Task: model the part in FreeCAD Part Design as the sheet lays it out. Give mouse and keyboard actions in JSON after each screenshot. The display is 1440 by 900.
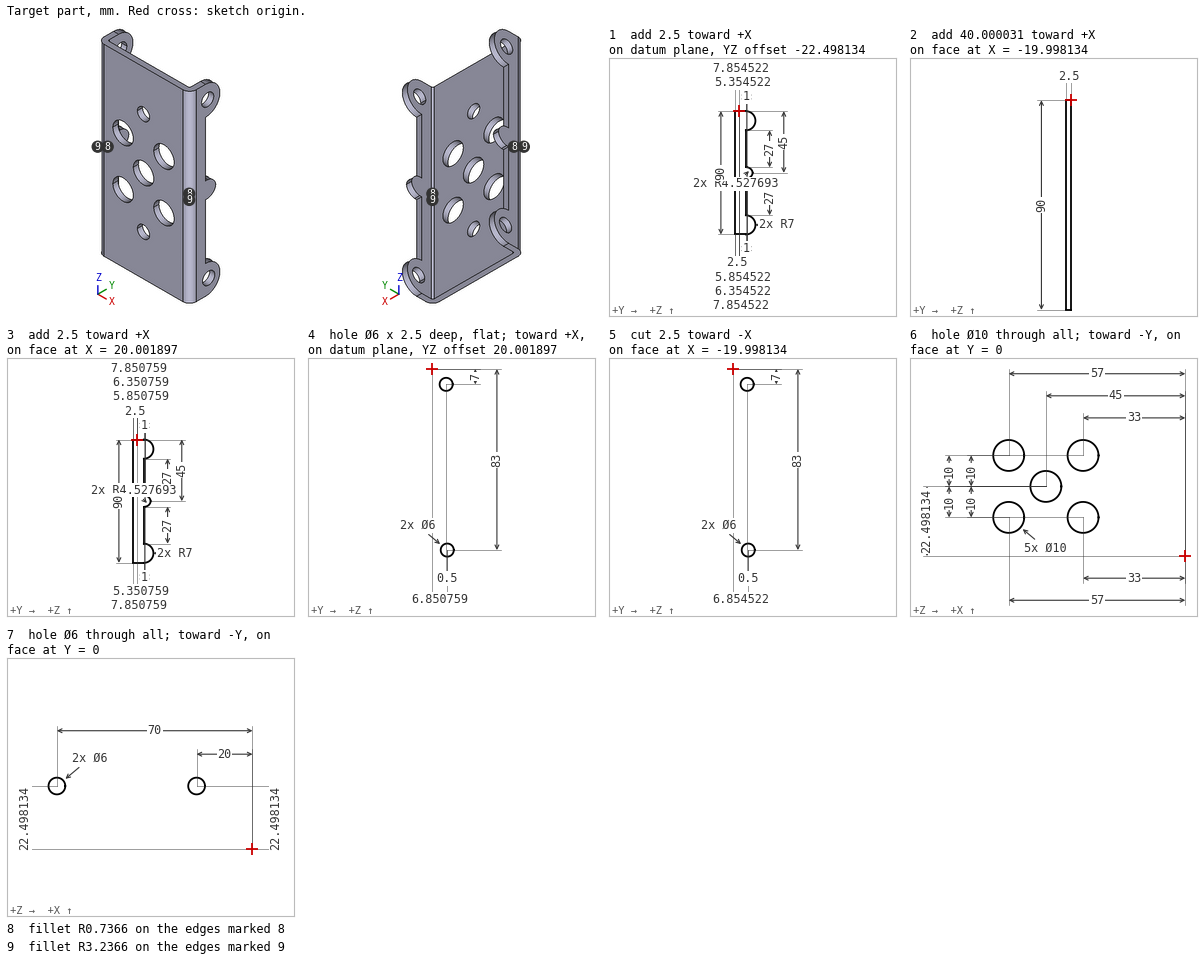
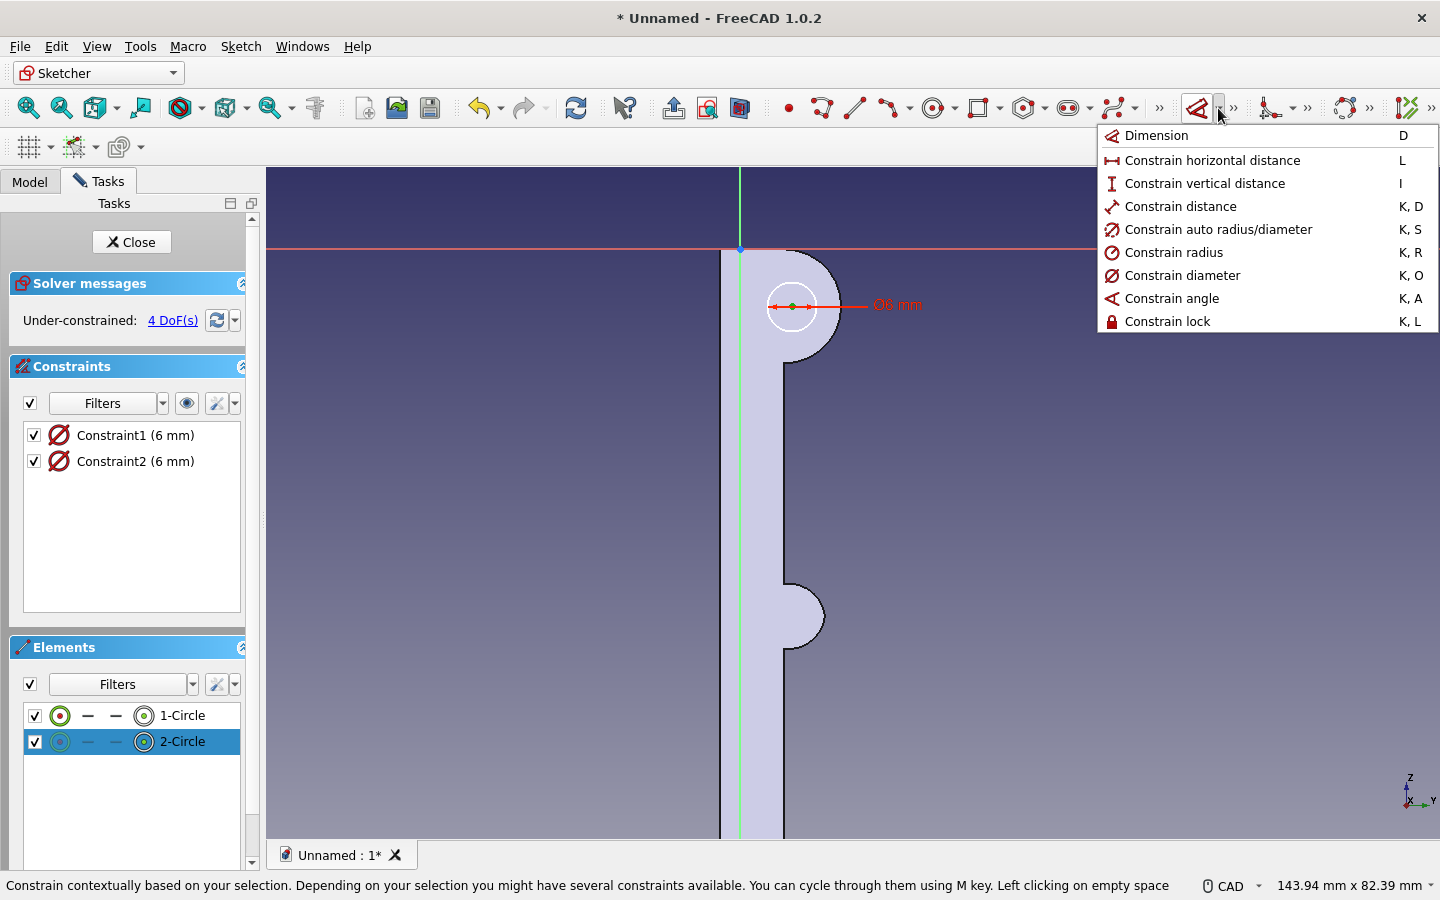
{"action": "left_click", "coordinate": [1268, 184]}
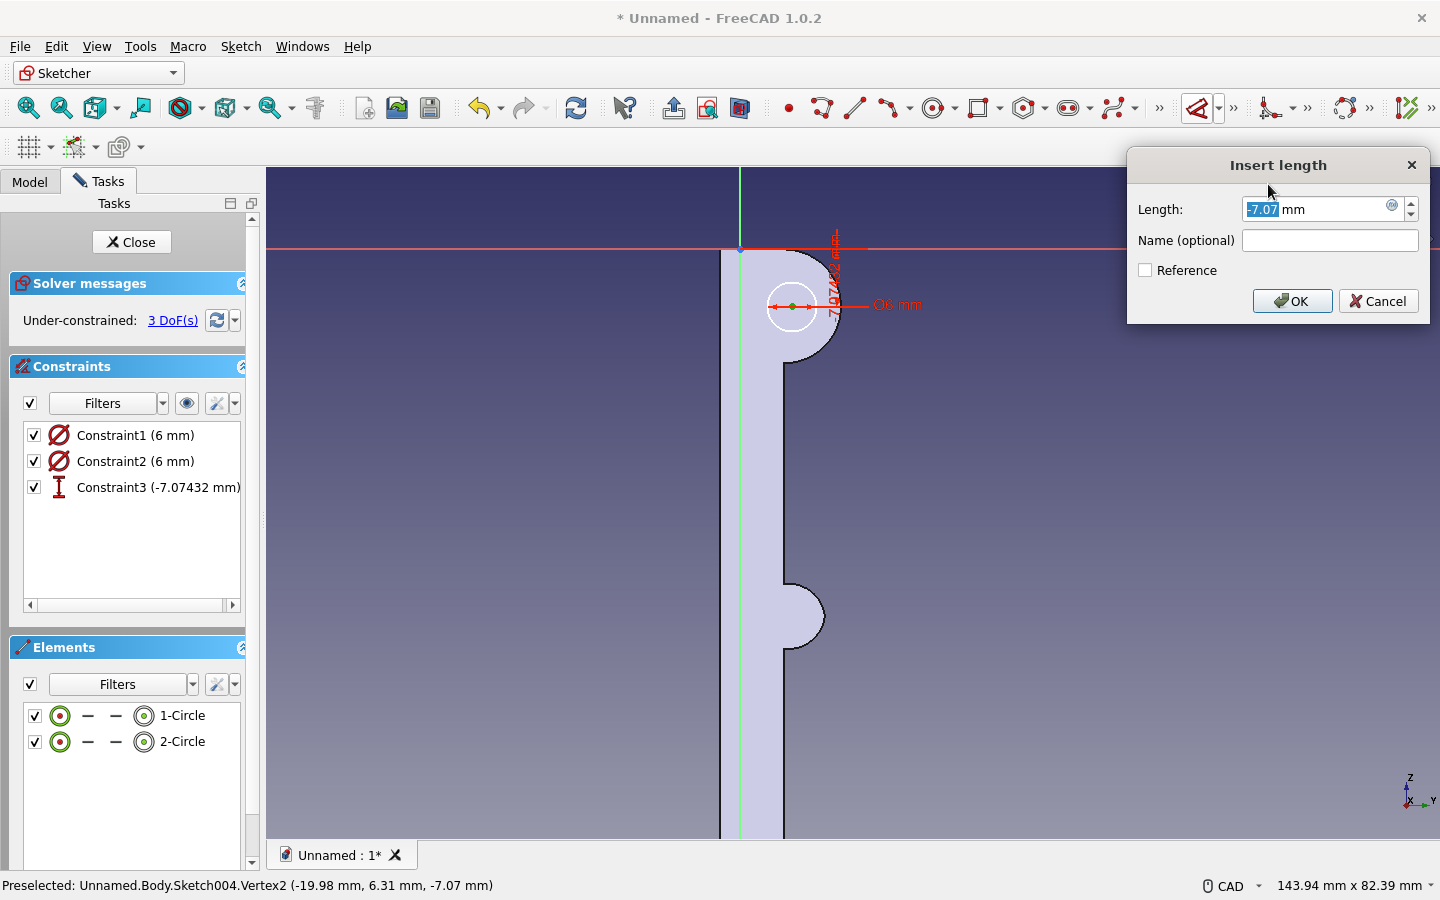
{"action": "type", "text": "-7"}
{"action": "key", "text": "Return"}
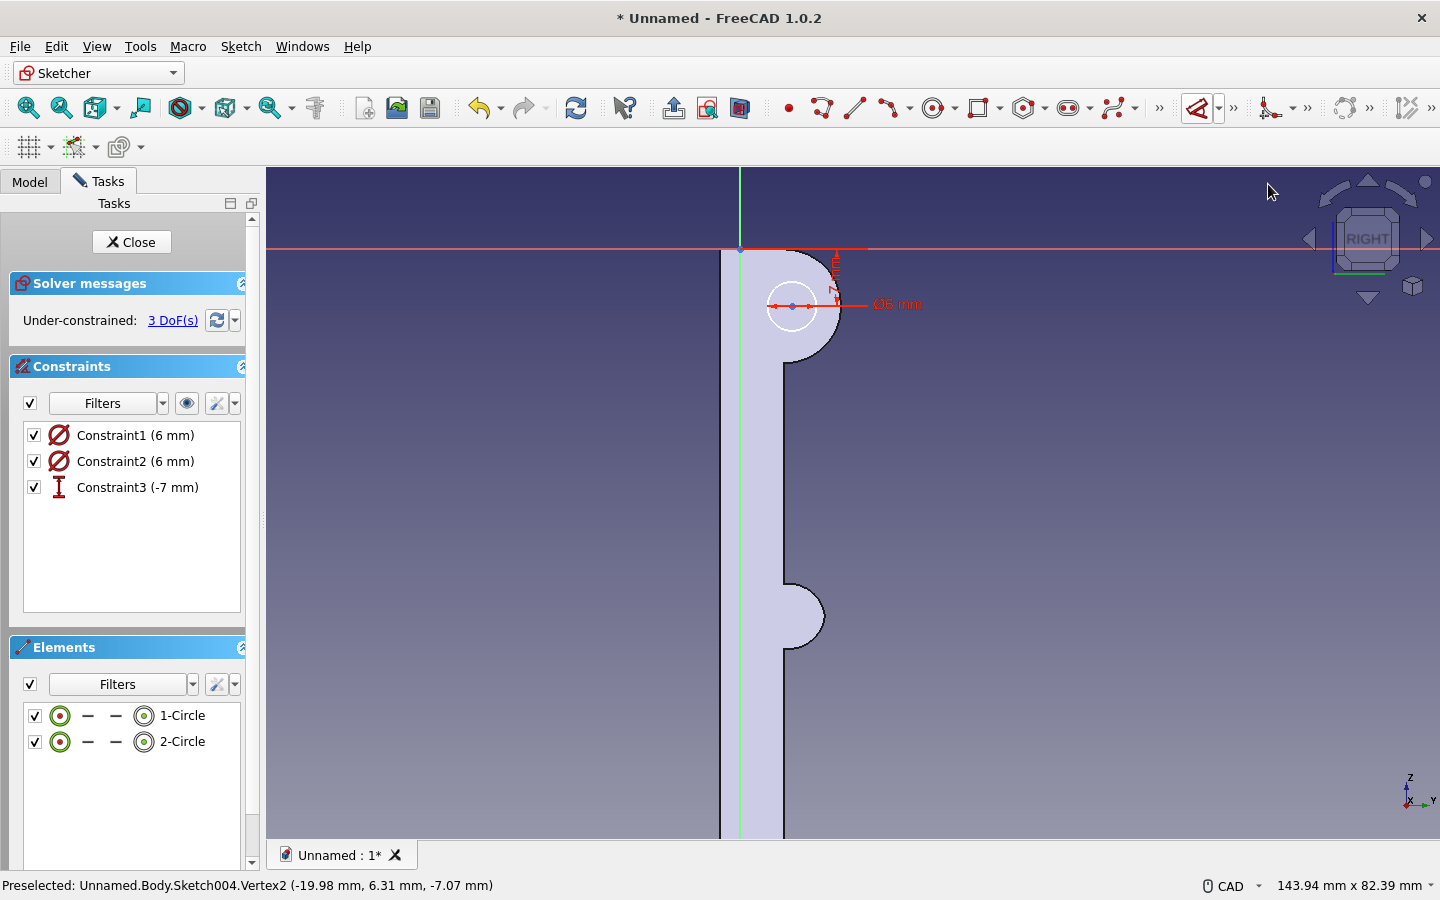
{"action": "scroll", "coordinate": [792, 306], "scroll_direction": "down", "scroll_amount": 2}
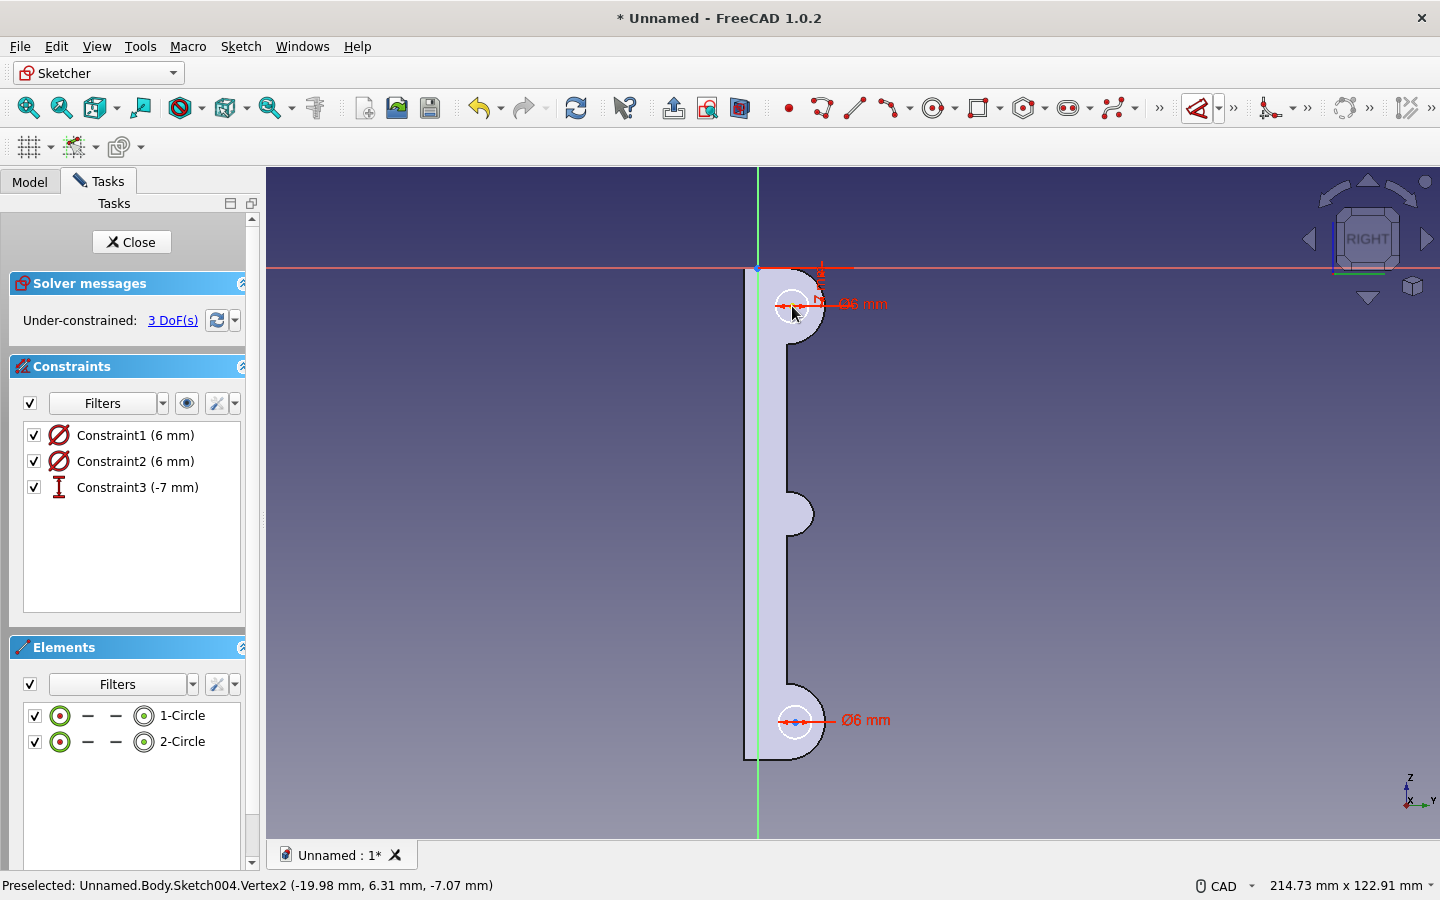
{"action": "left_click", "coordinate": [795, 722]}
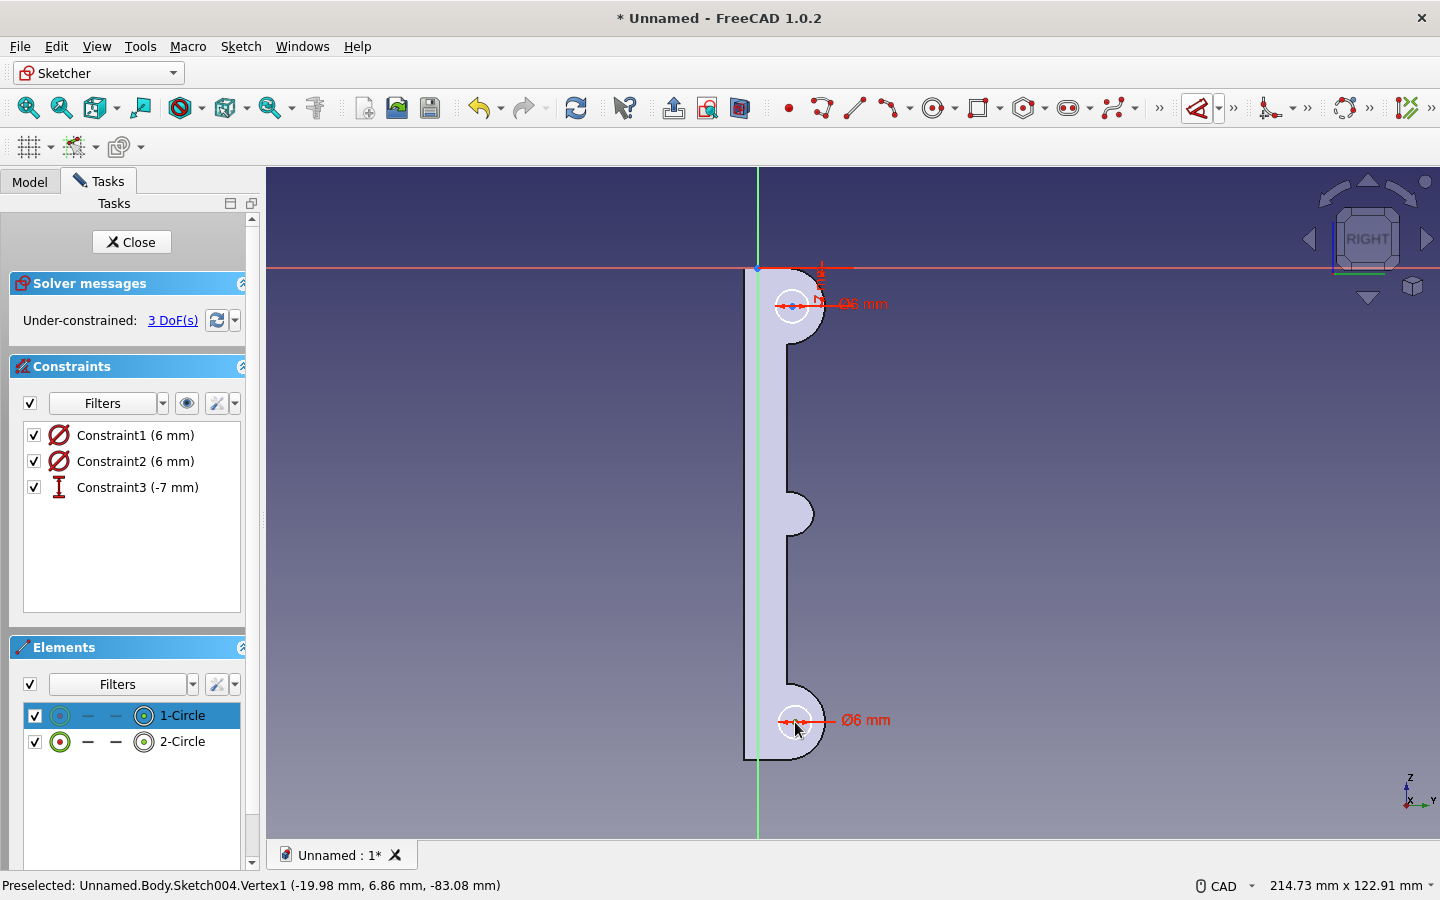
{"action": "key", "text": "i"}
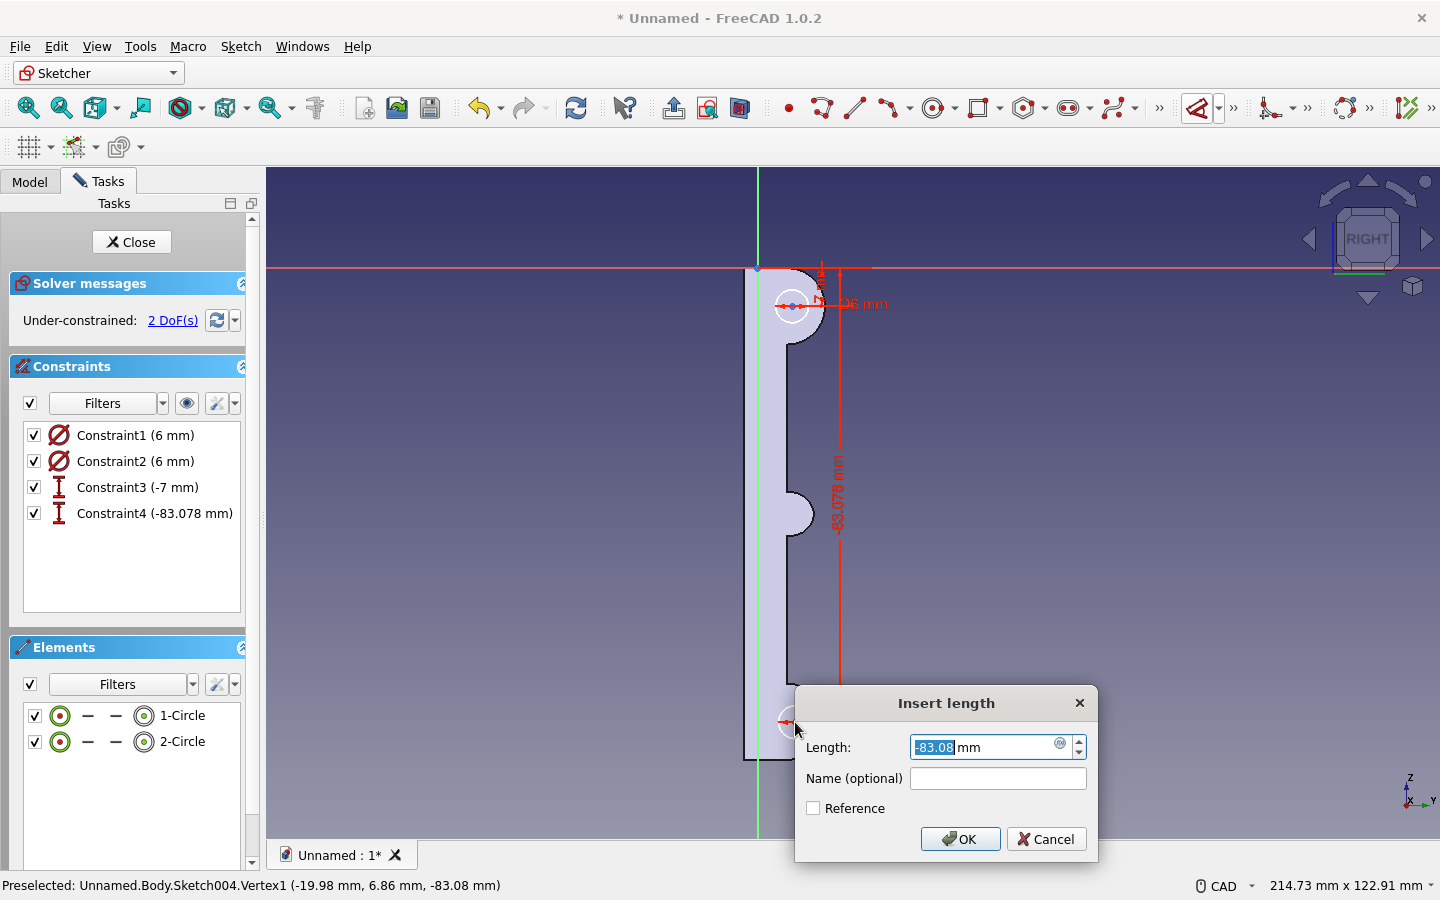
{"action": "type", "text": "-83"}
{"action": "key", "text": "Return"}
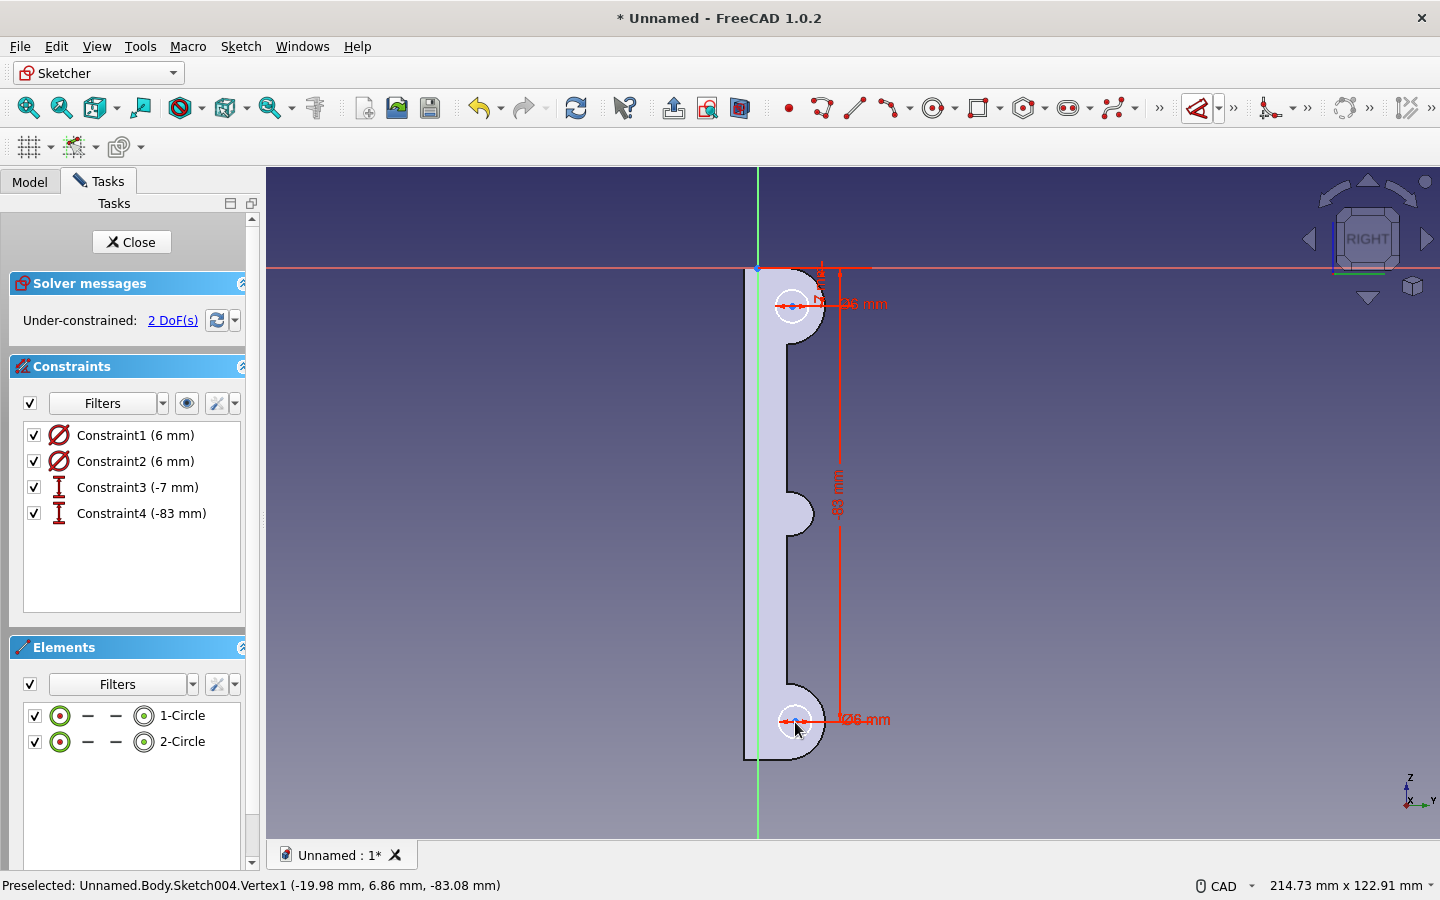
{"action": "scroll", "coordinate": [795, 722], "scroll_direction": "up", "scroll_amount": 14}